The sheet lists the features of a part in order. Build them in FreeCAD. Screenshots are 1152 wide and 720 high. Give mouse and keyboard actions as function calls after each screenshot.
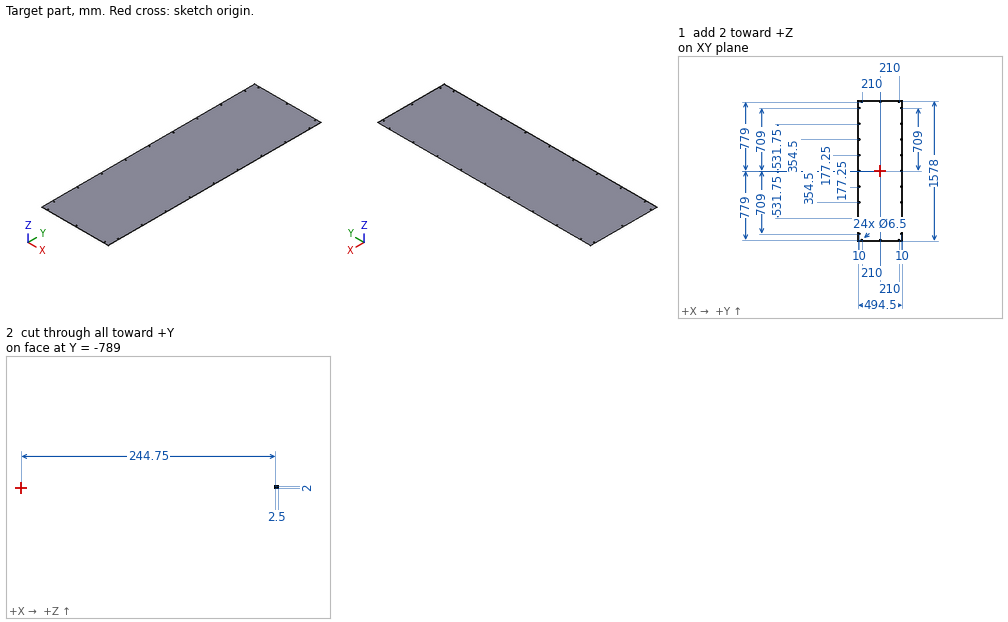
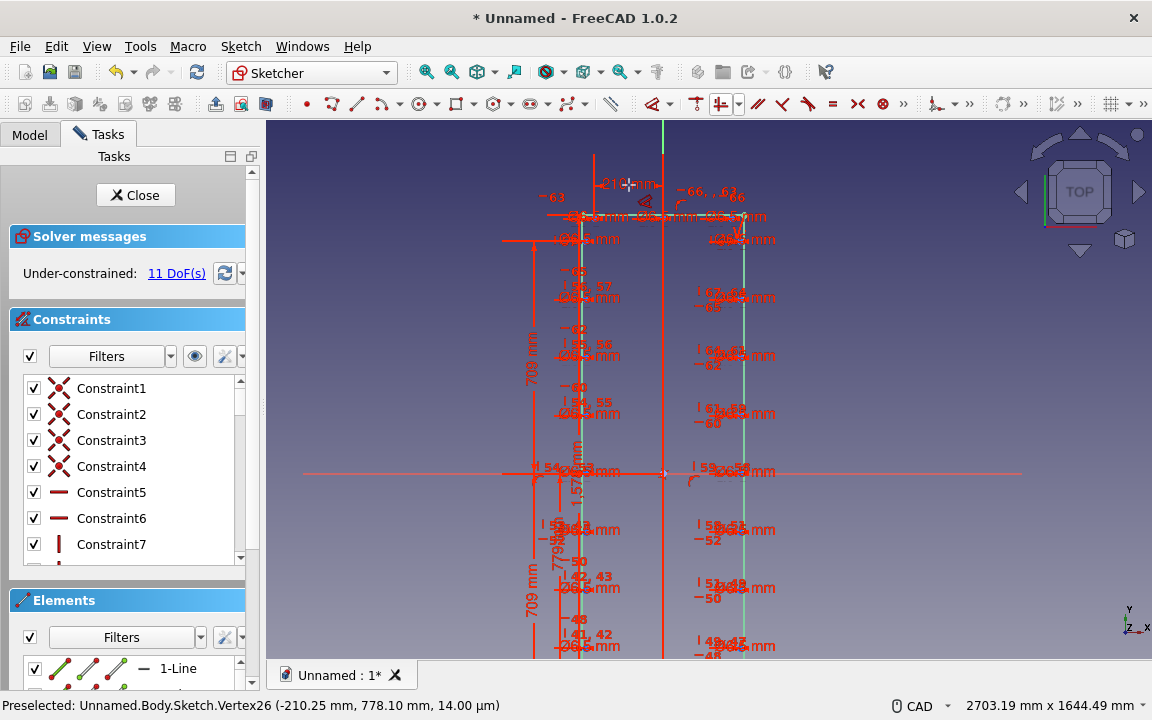
click(594, 219)
click(560, 288)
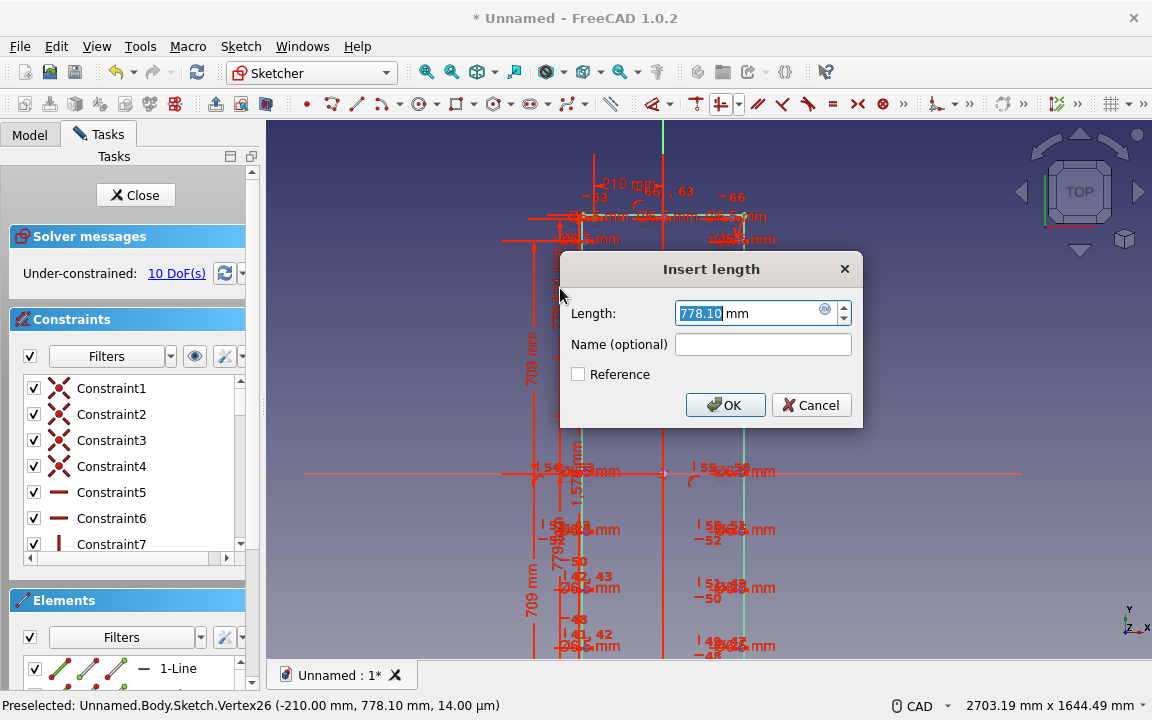
text(779)
key(Return)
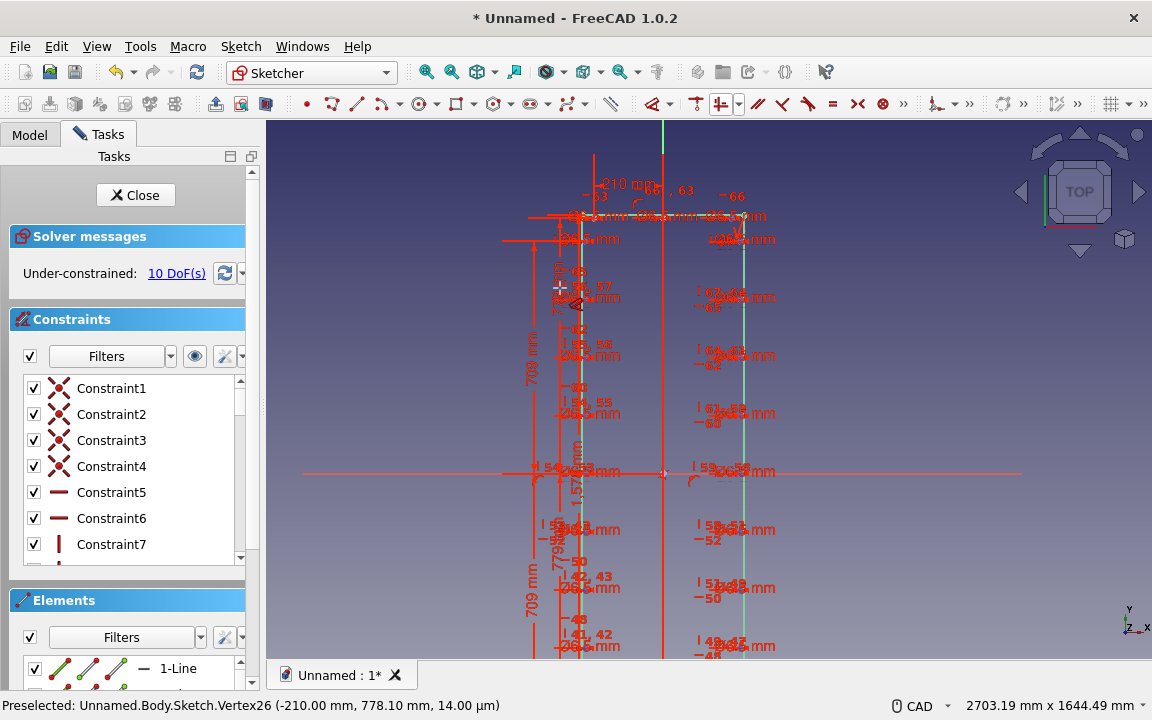
click(732, 218)
click(713, 184)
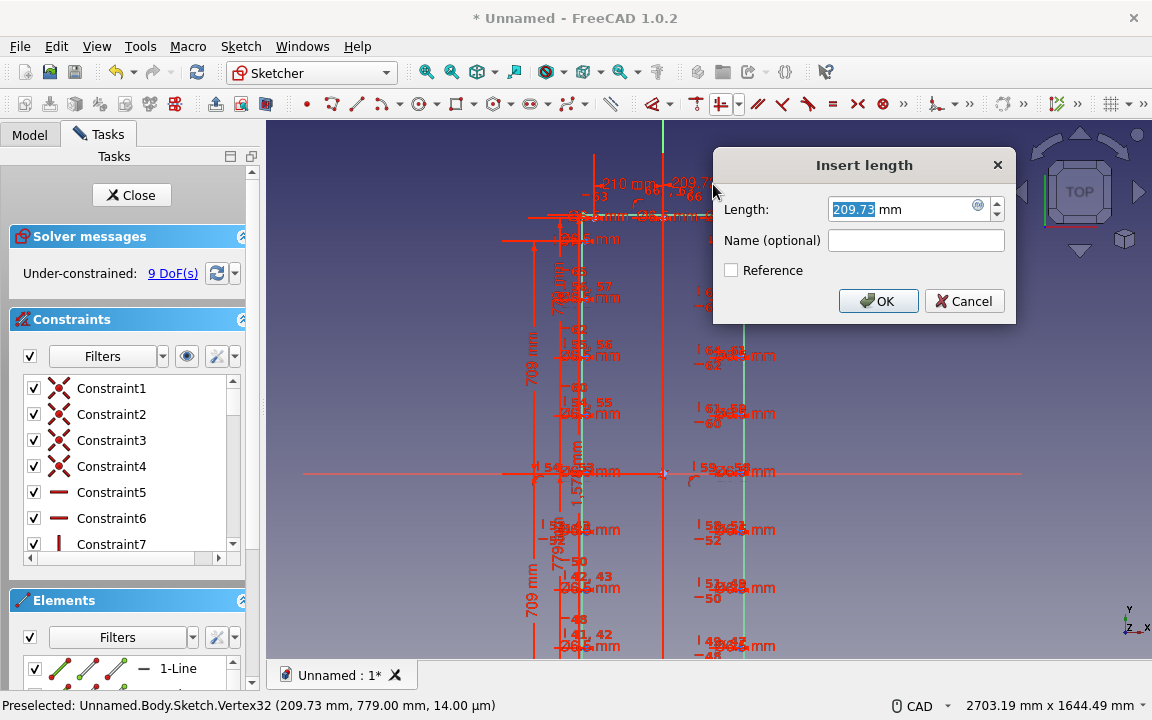
text(210)
key(Return)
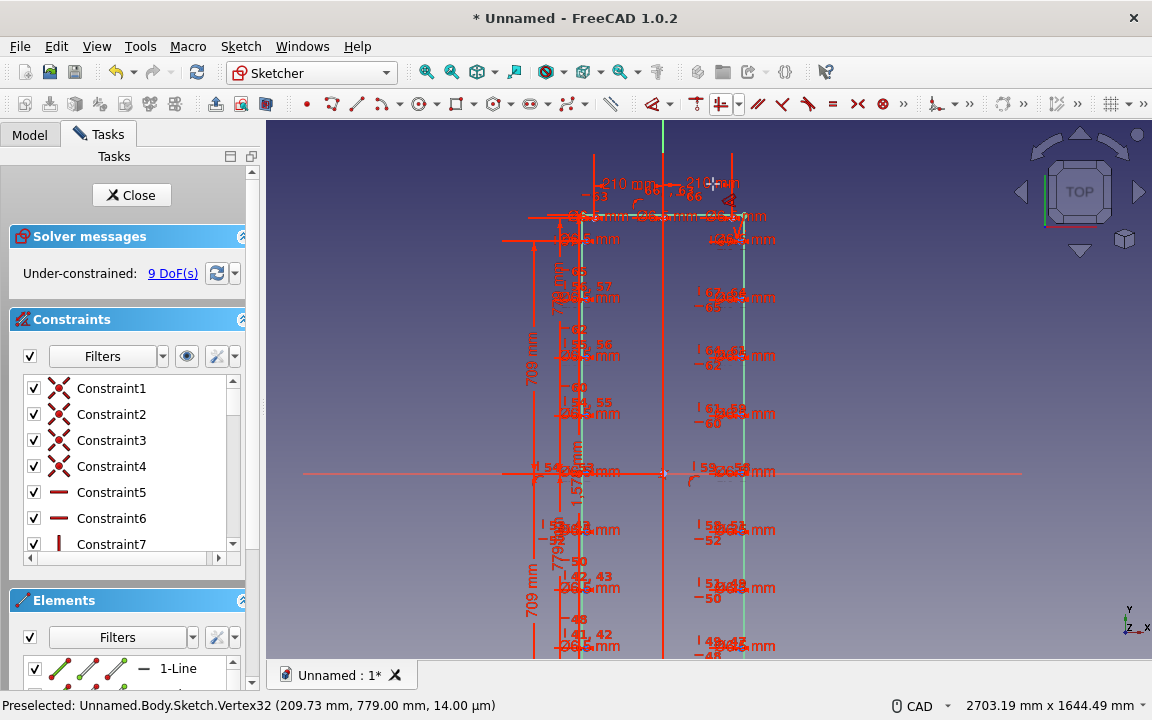
click(741, 242)
click(775, 358)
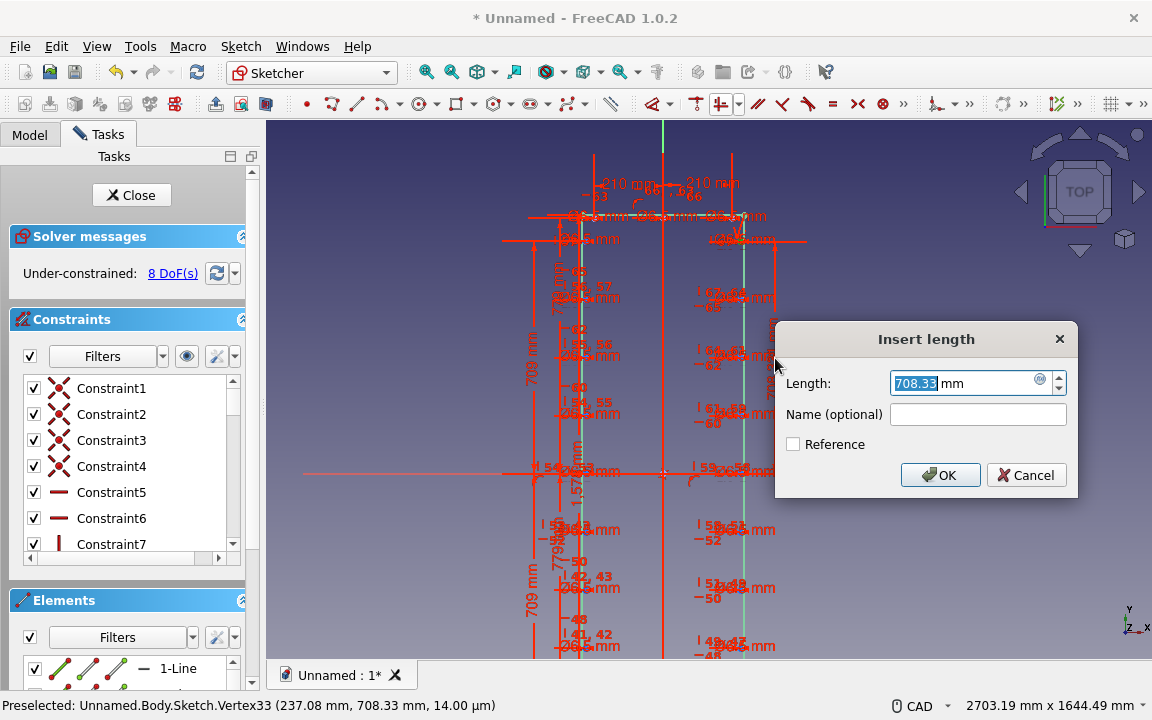
text(709)
key(Return)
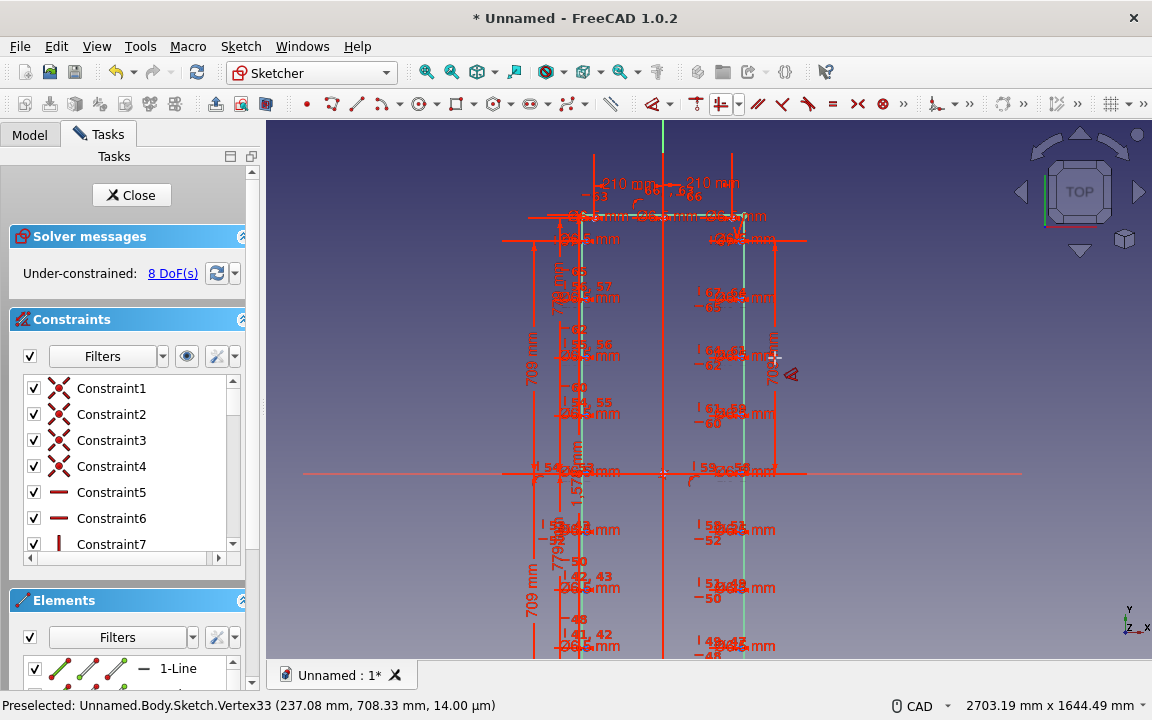
scroll(594, 218, down, 2)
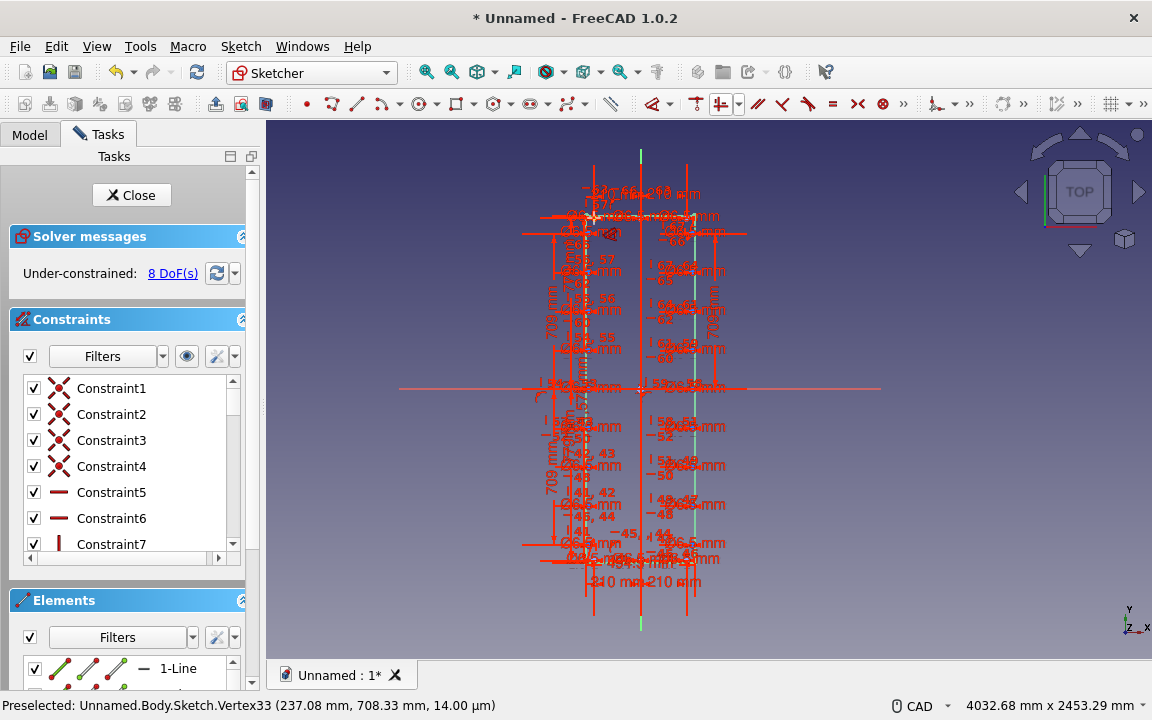
scroll(586, 563, up, 15)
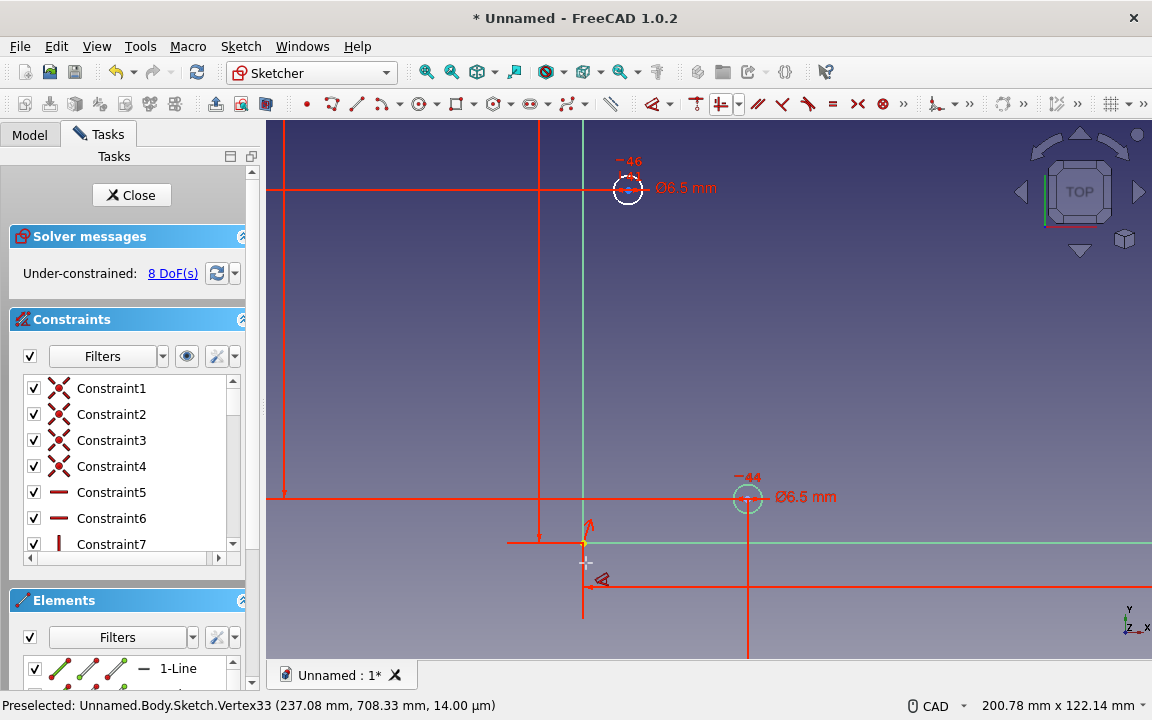
click(583, 543)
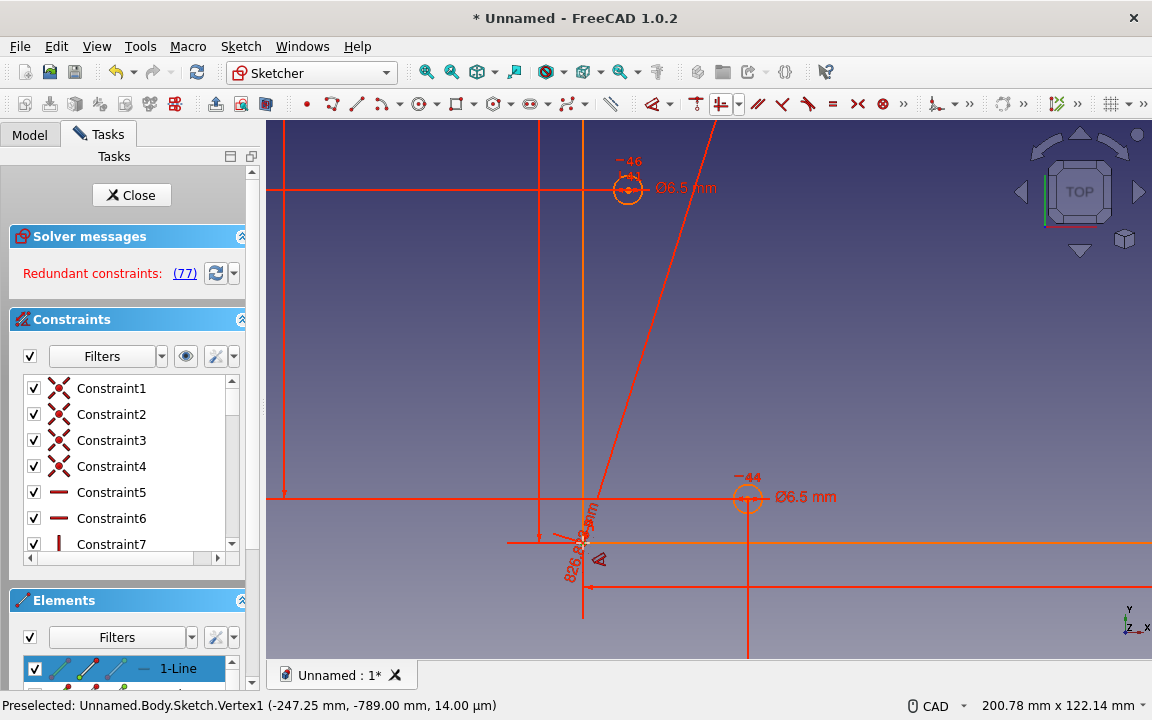
click(628, 190)
click(606, 577)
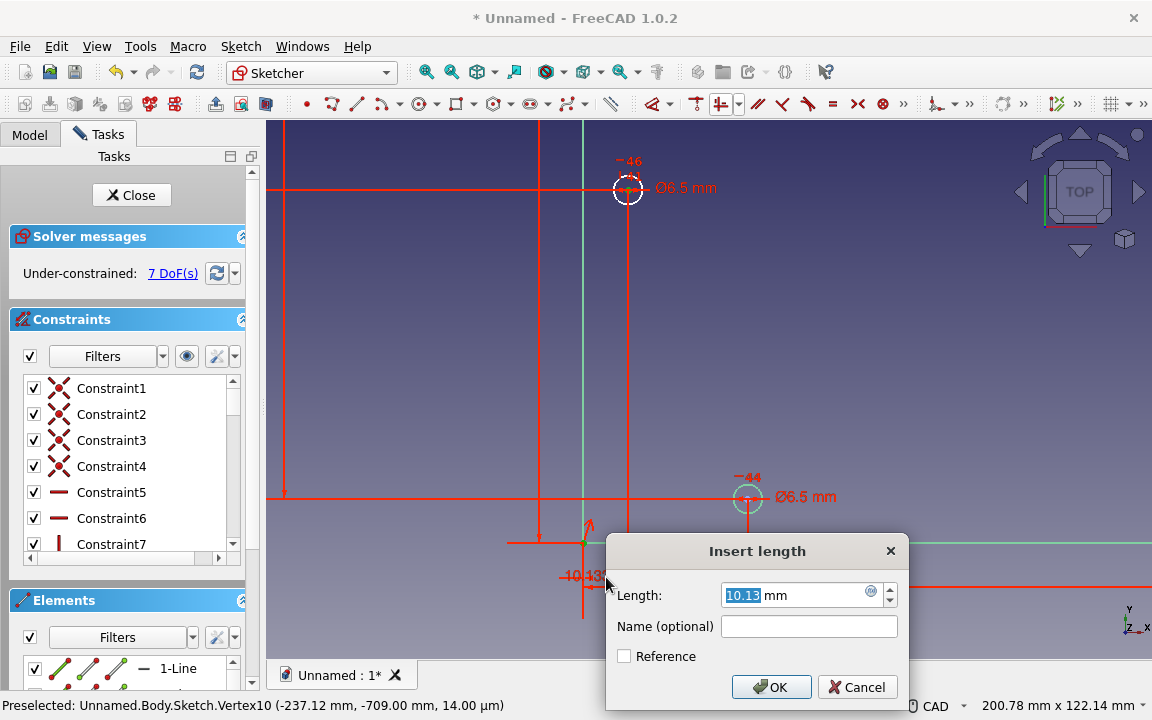
text(10)
key(Return)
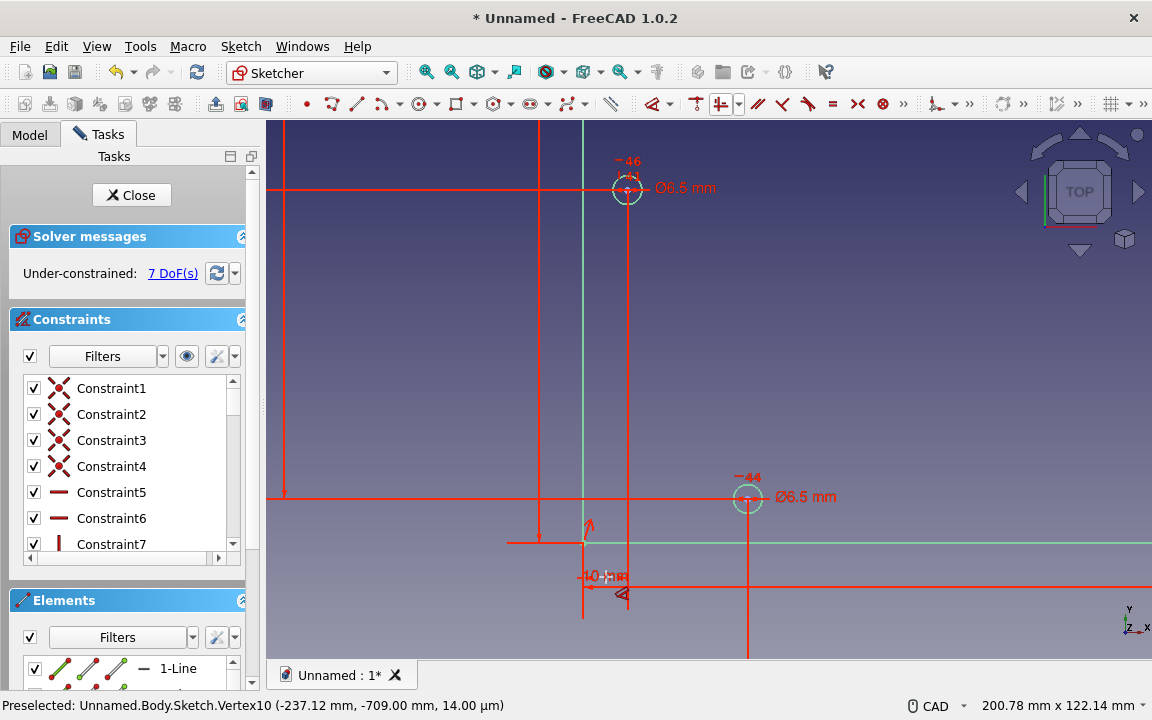
scroll(586, 564, down, 15)